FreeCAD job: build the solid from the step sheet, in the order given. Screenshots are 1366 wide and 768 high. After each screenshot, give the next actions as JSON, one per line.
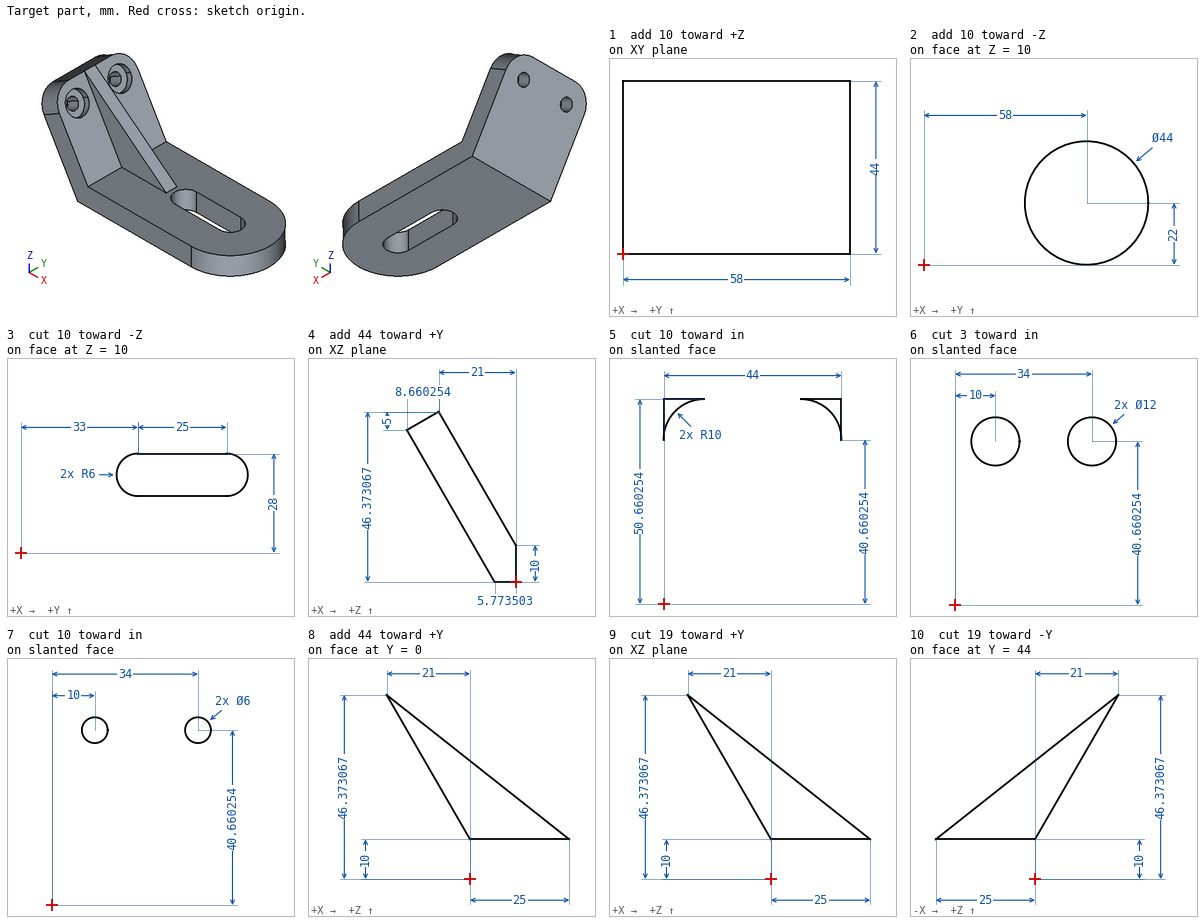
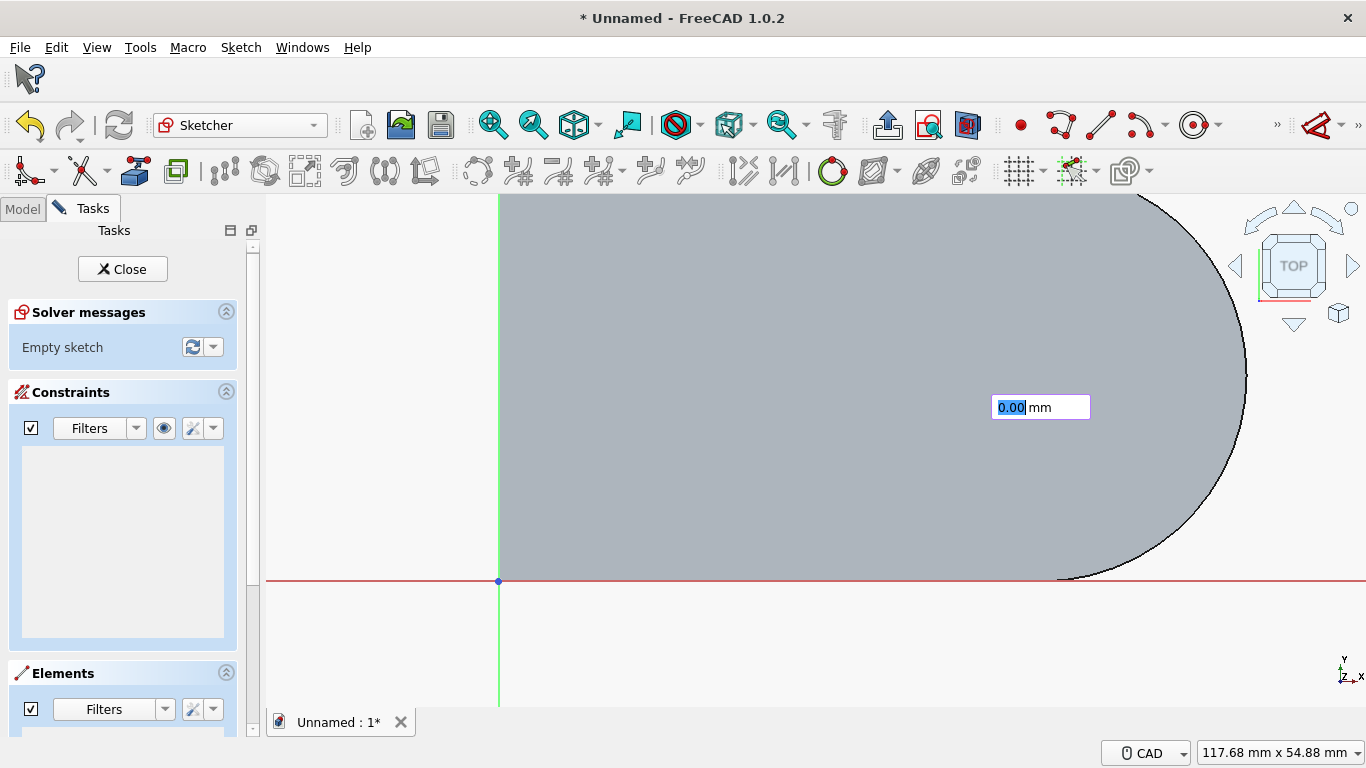
{"action": "left_click", "coordinate": [924, 320]}
{"action": "key", "text": "Escape"}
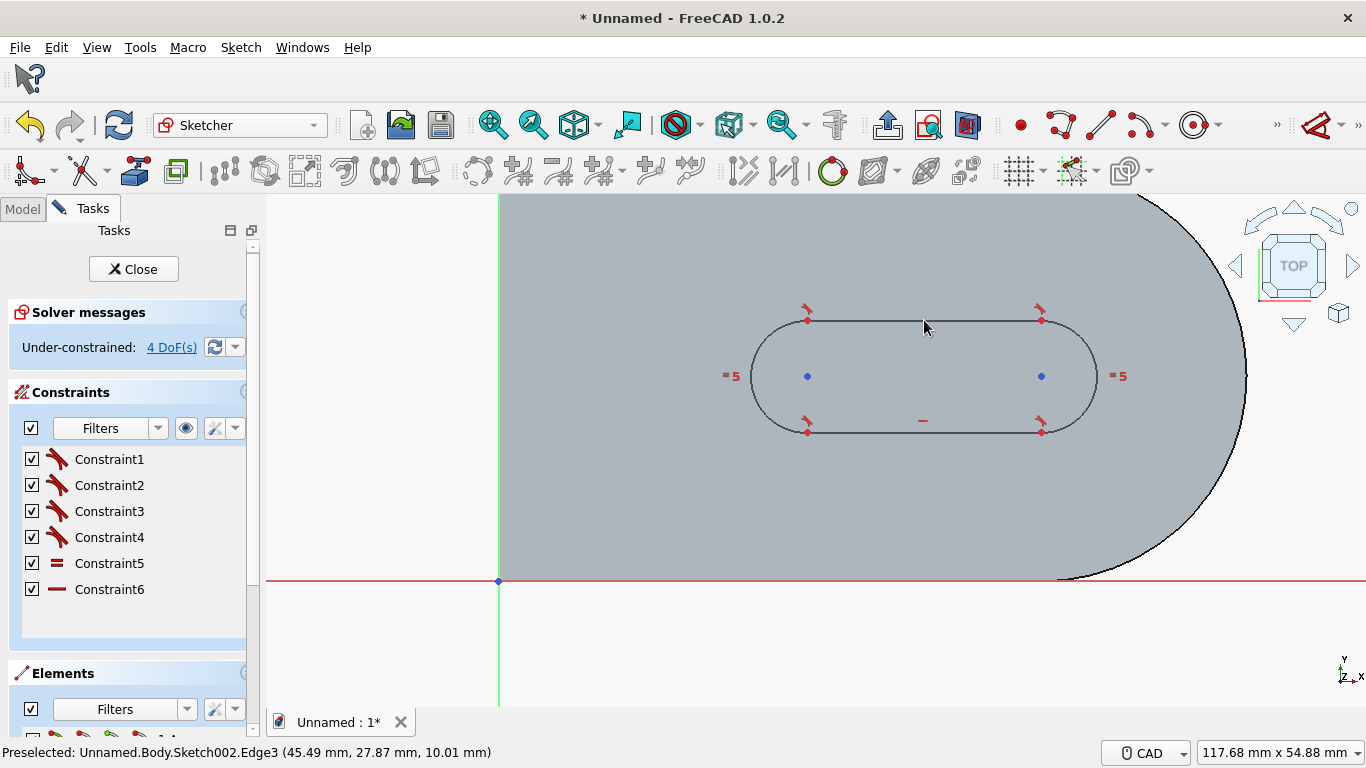
{"action": "left_click", "coordinate": [1316, 126]}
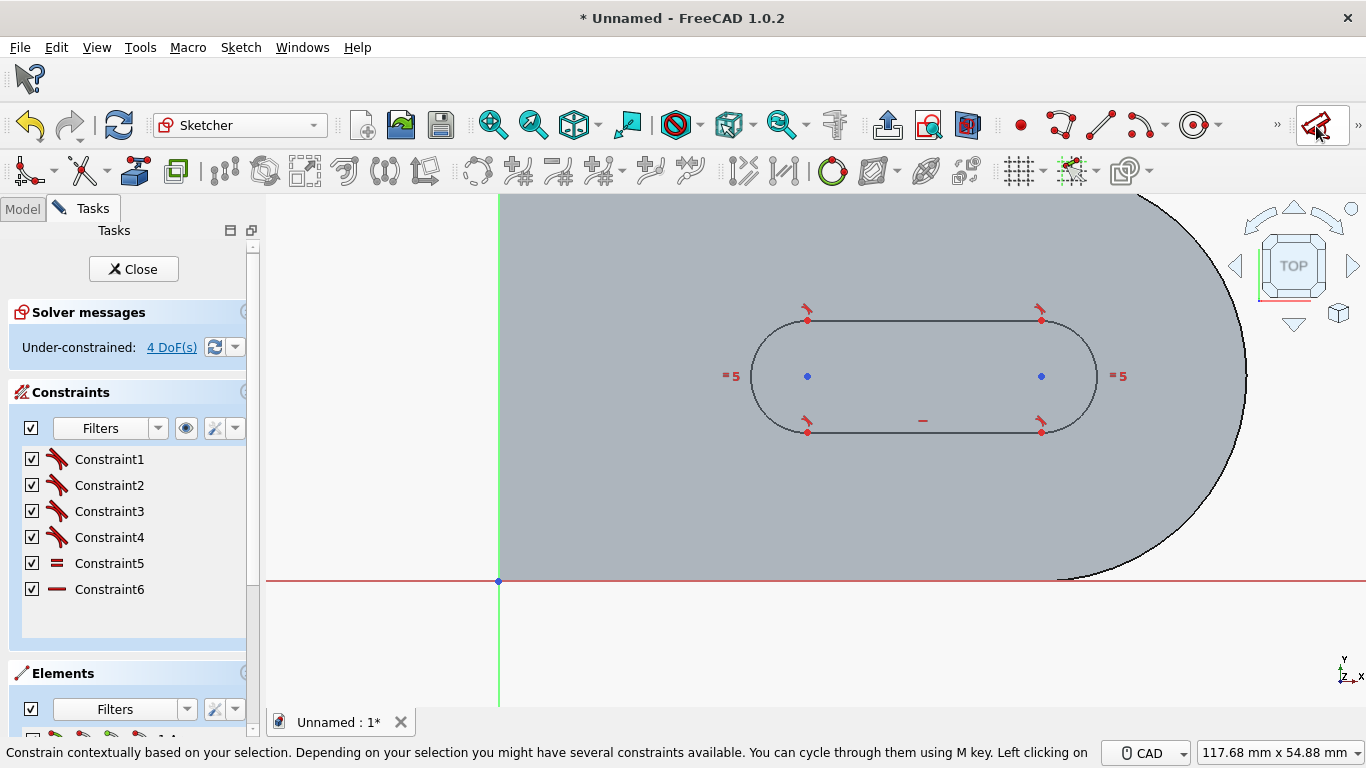
{"action": "left_click", "coordinate": [762, 344]}
{"action": "left_click", "coordinate": [736, 325]}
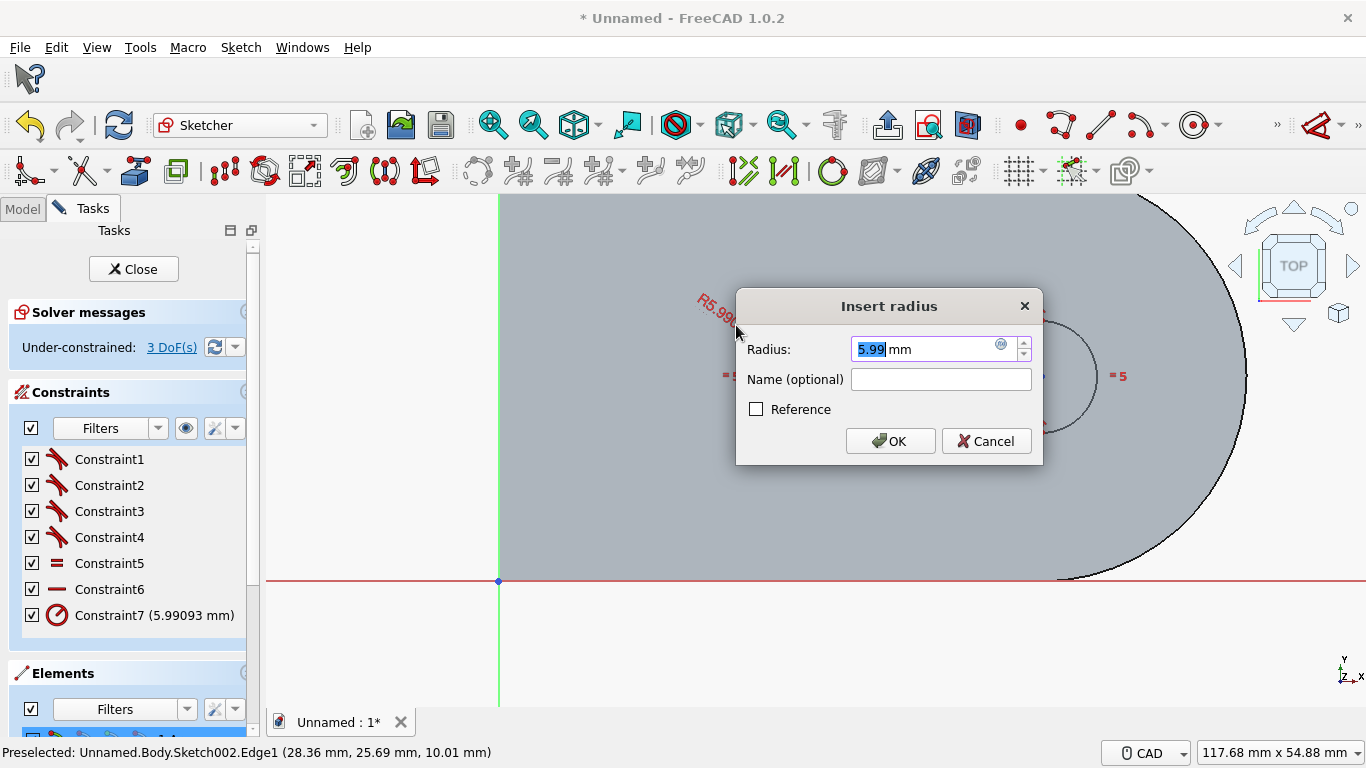
{"action": "type", "text": "6"}
{"action": "key", "text": "Return"}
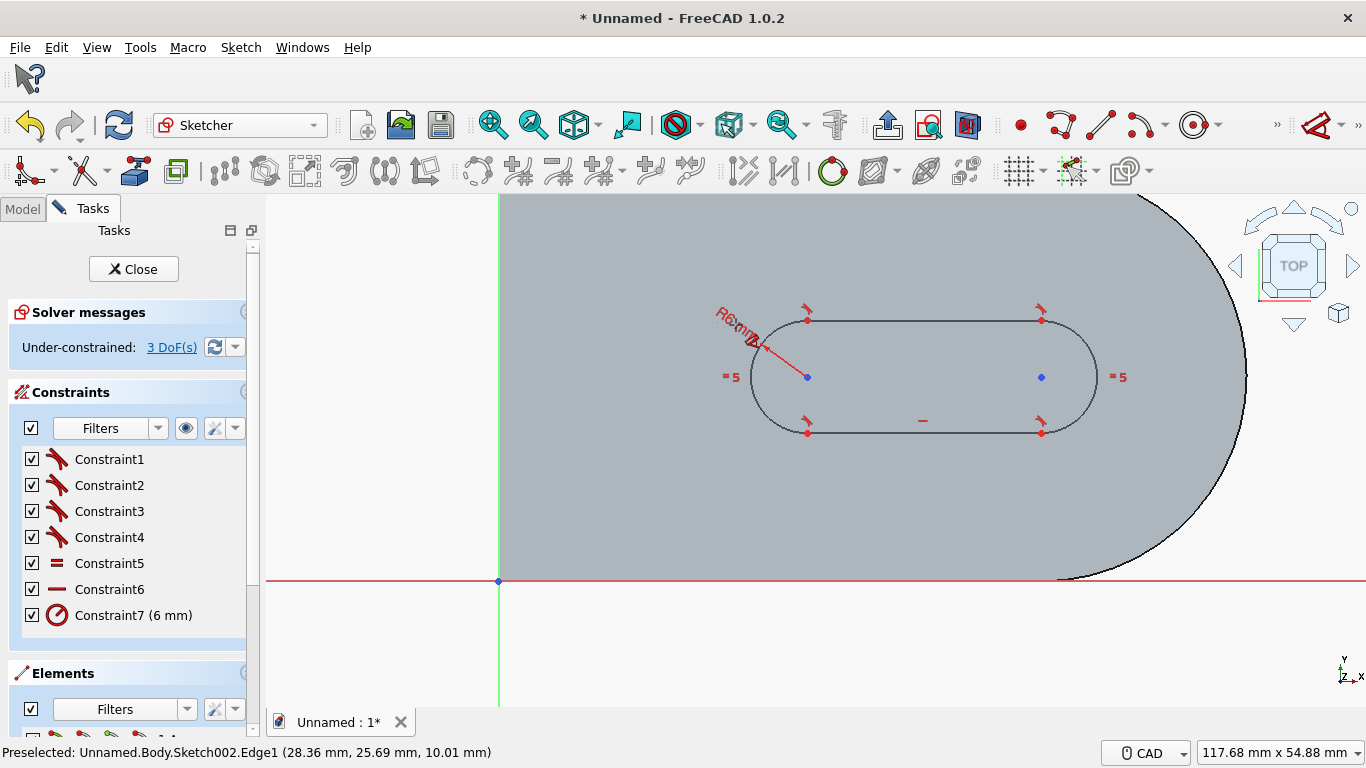
{"action": "left_click", "coordinate": [877, 321]}
{"action": "left_click", "coordinate": [924, 287]}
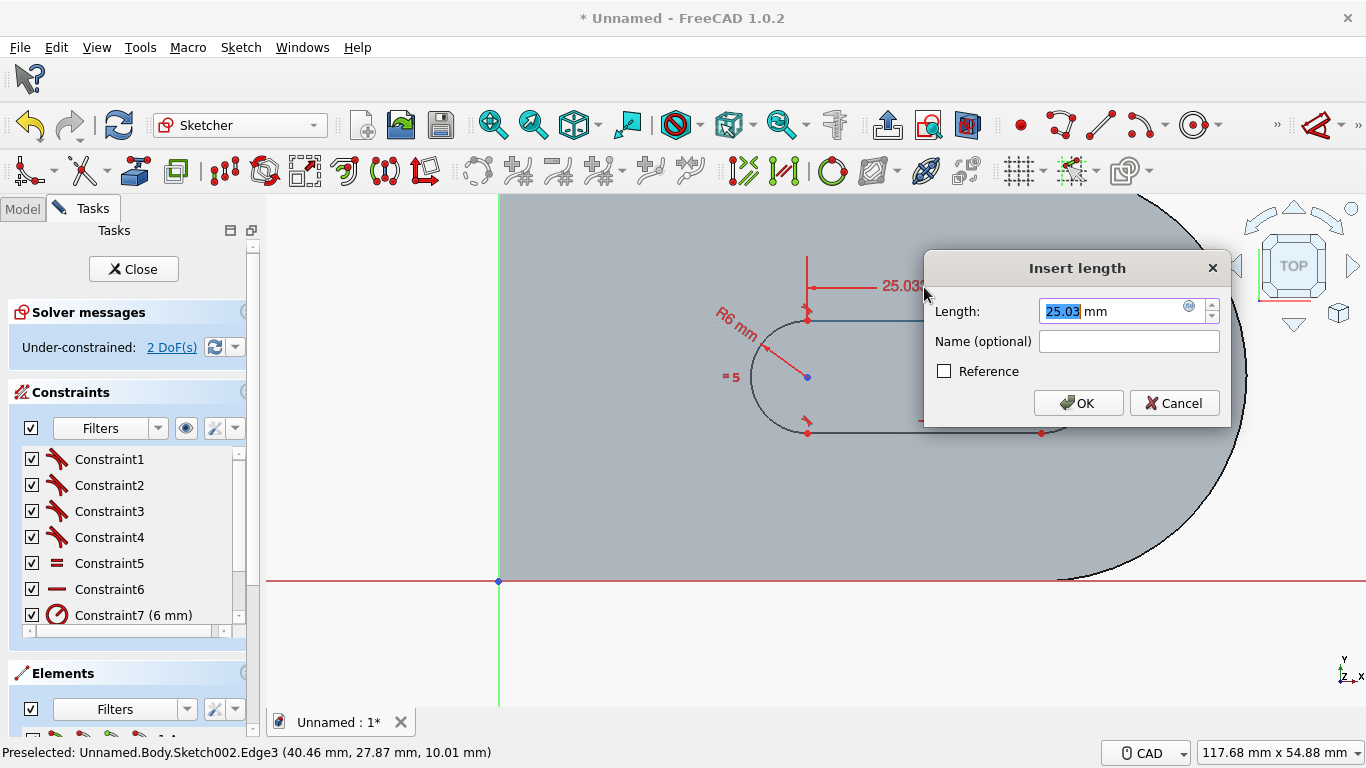
{"action": "type", "text": "25"}
{"action": "key", "text": "Return"}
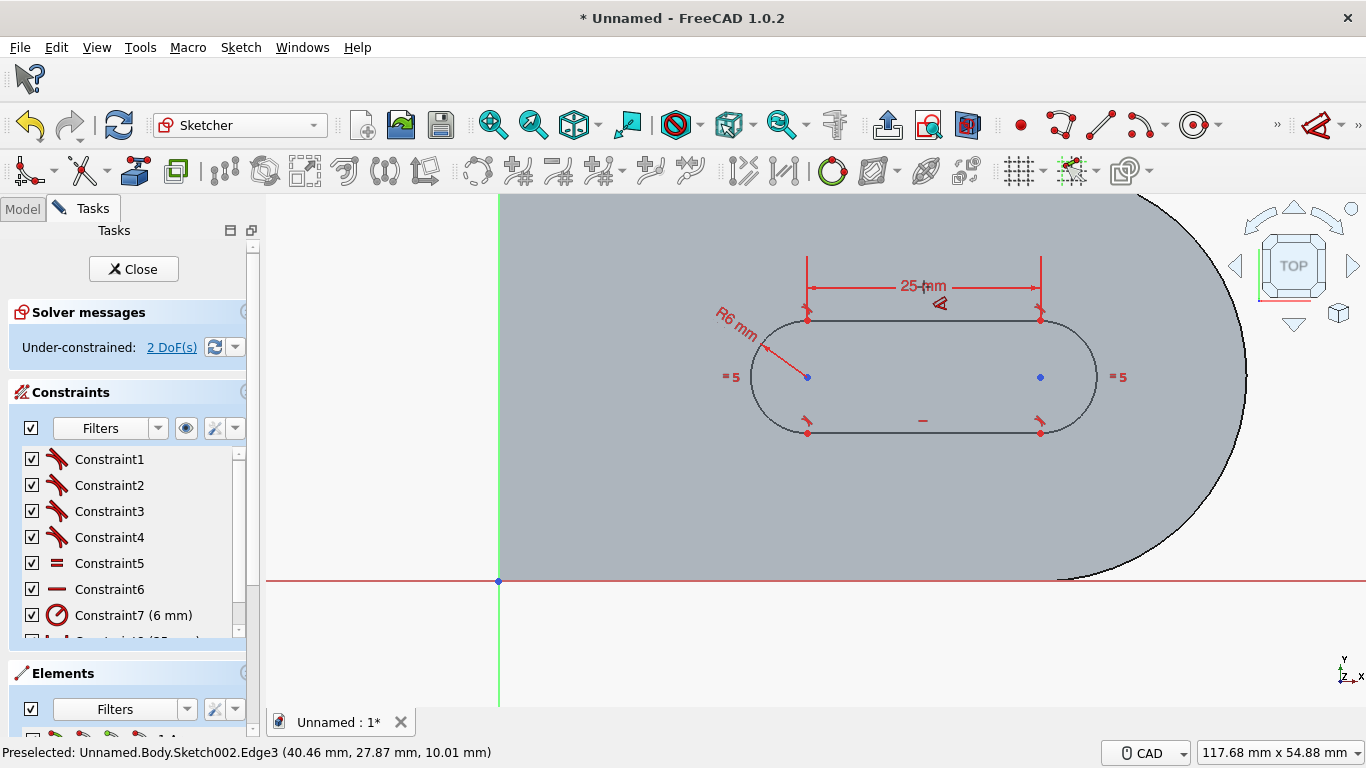
{"action": "left_click", "coordinate": [807, 321]}
{"action": "left_click", "coordinate": [653, 615]}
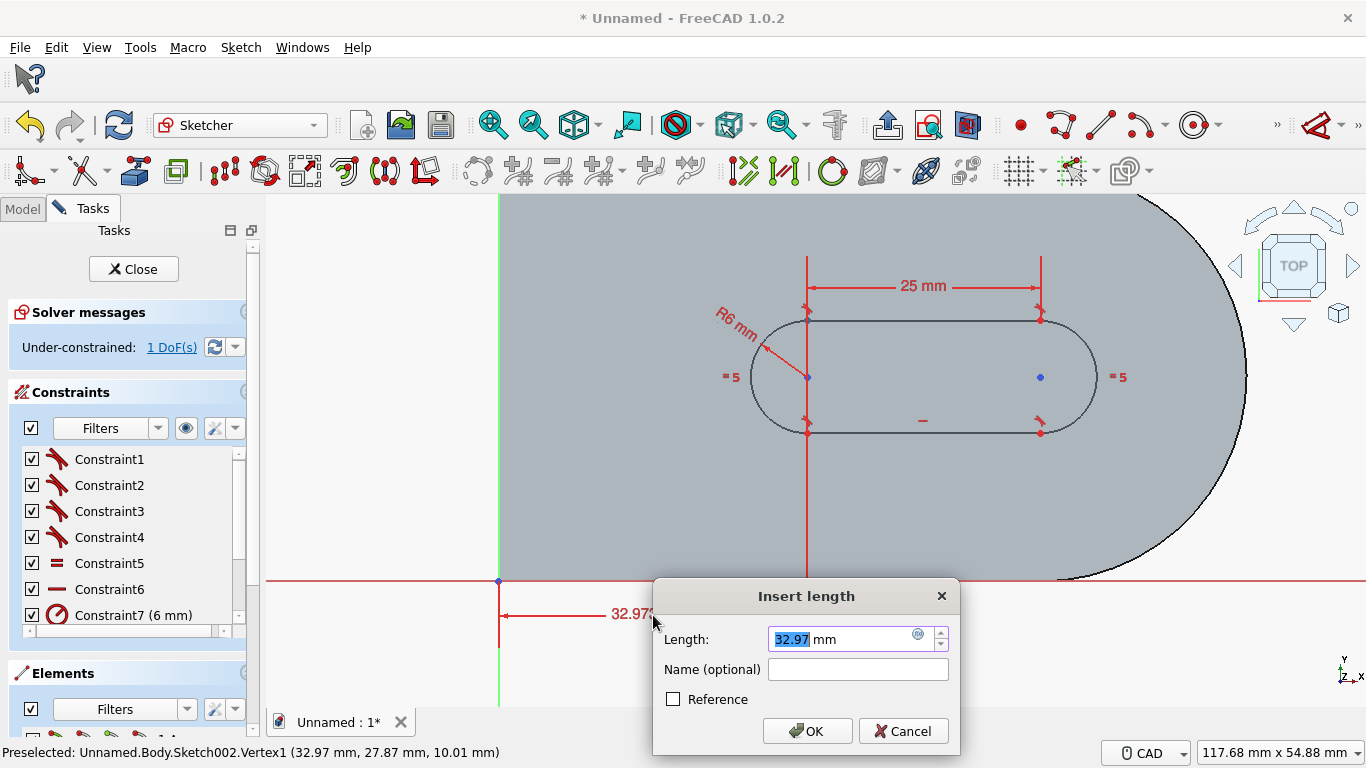
{"action": "type", "text": "33"}
{"action": "key", "text": "Return"}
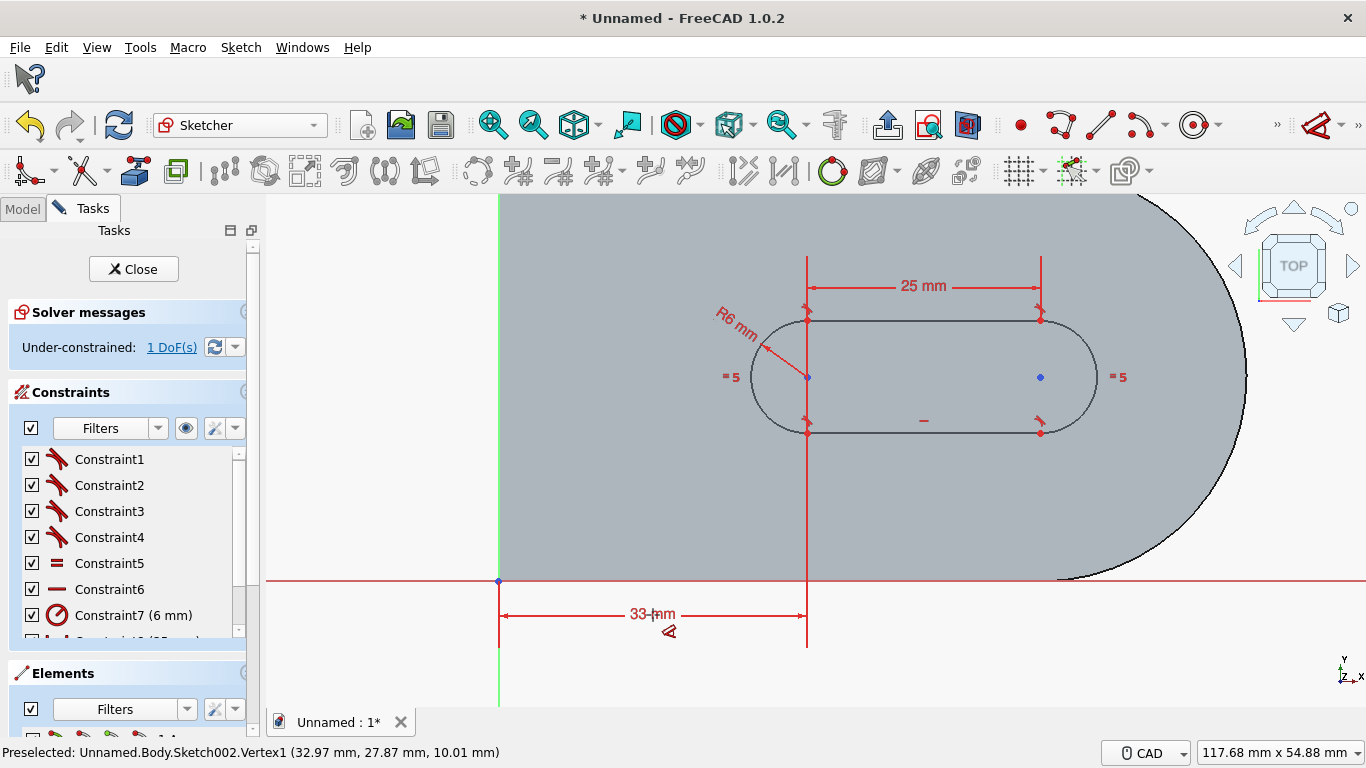
{"action": "left_click", "coordinate": [807, 321]}
{"action": "left_click", "coordinate": [465, 451]}